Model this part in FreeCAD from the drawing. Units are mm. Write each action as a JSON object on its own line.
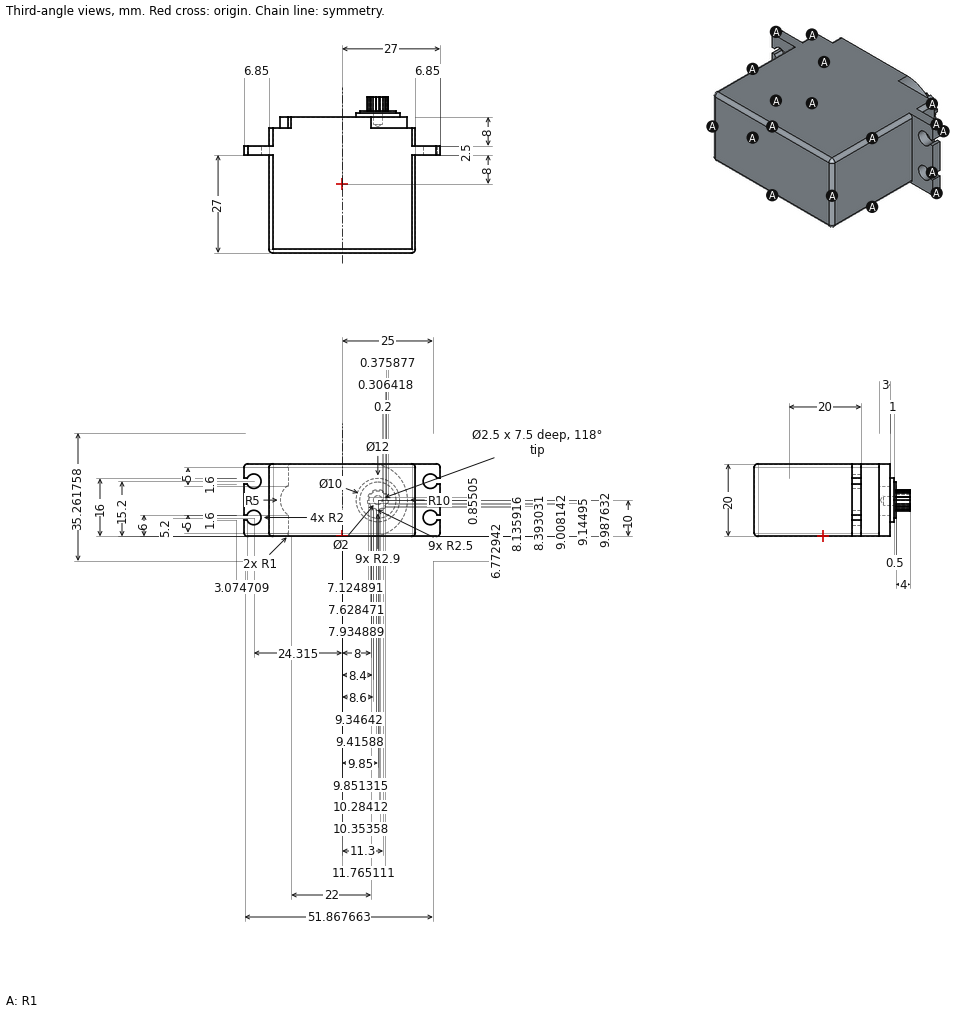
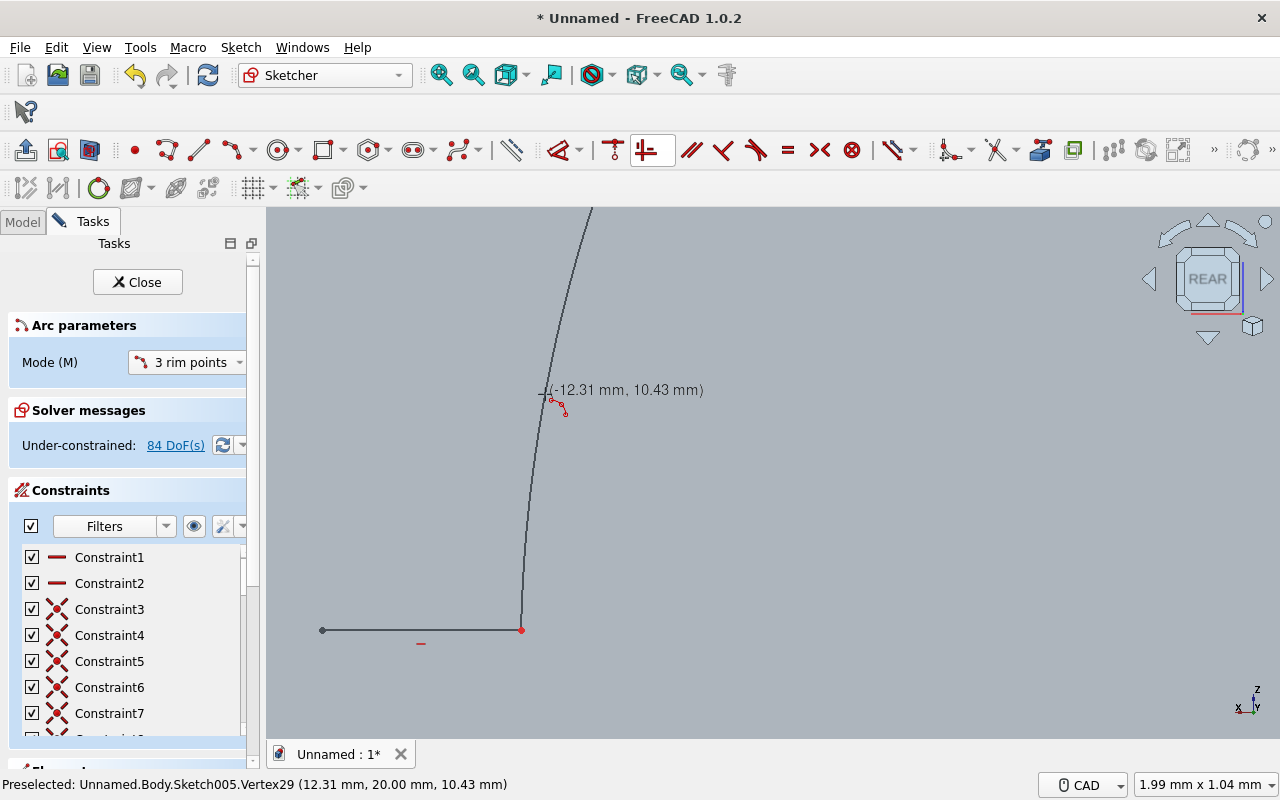
{"action": "scroll", "coordinate": [554, 370], "scroll_direction": "down", "scroll_amount": 15}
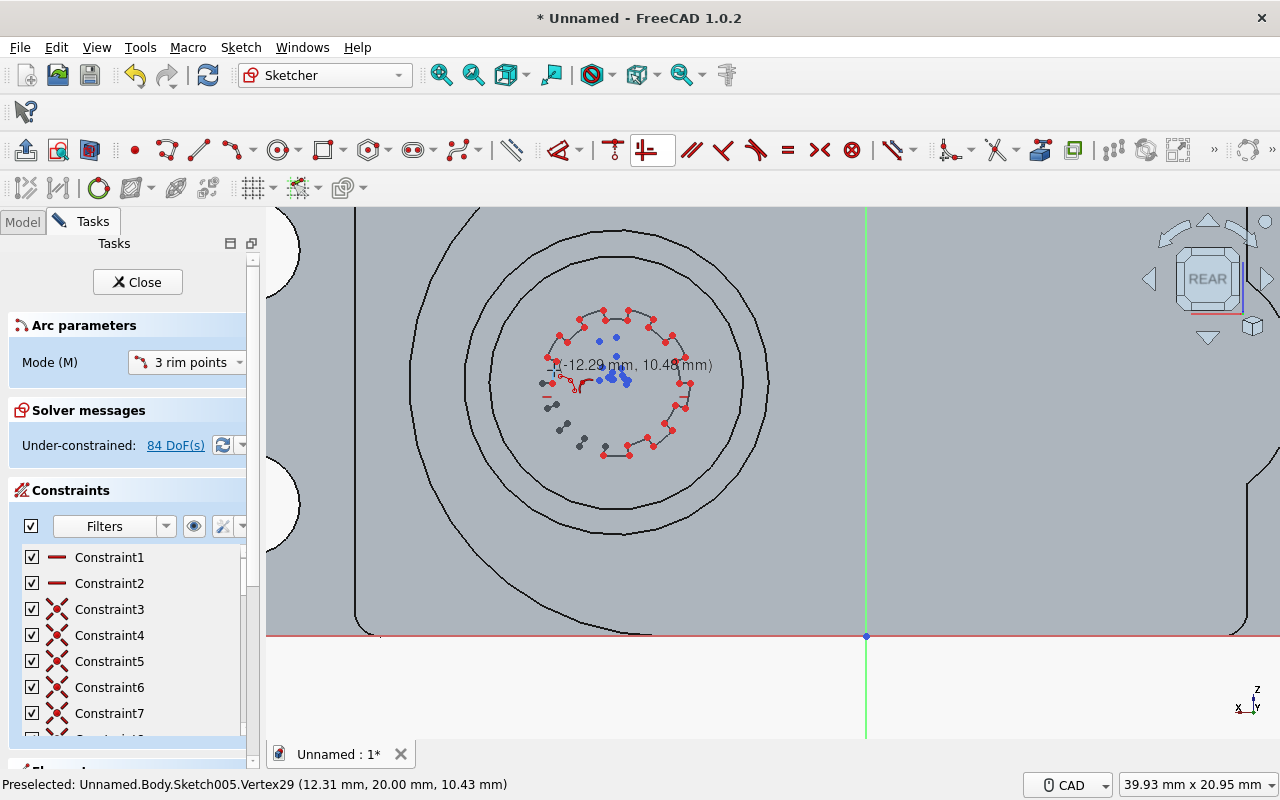
{"action": "scroll", "coordinate": [543, 383], "scroll_direction": "up", "scroll_amount": 6}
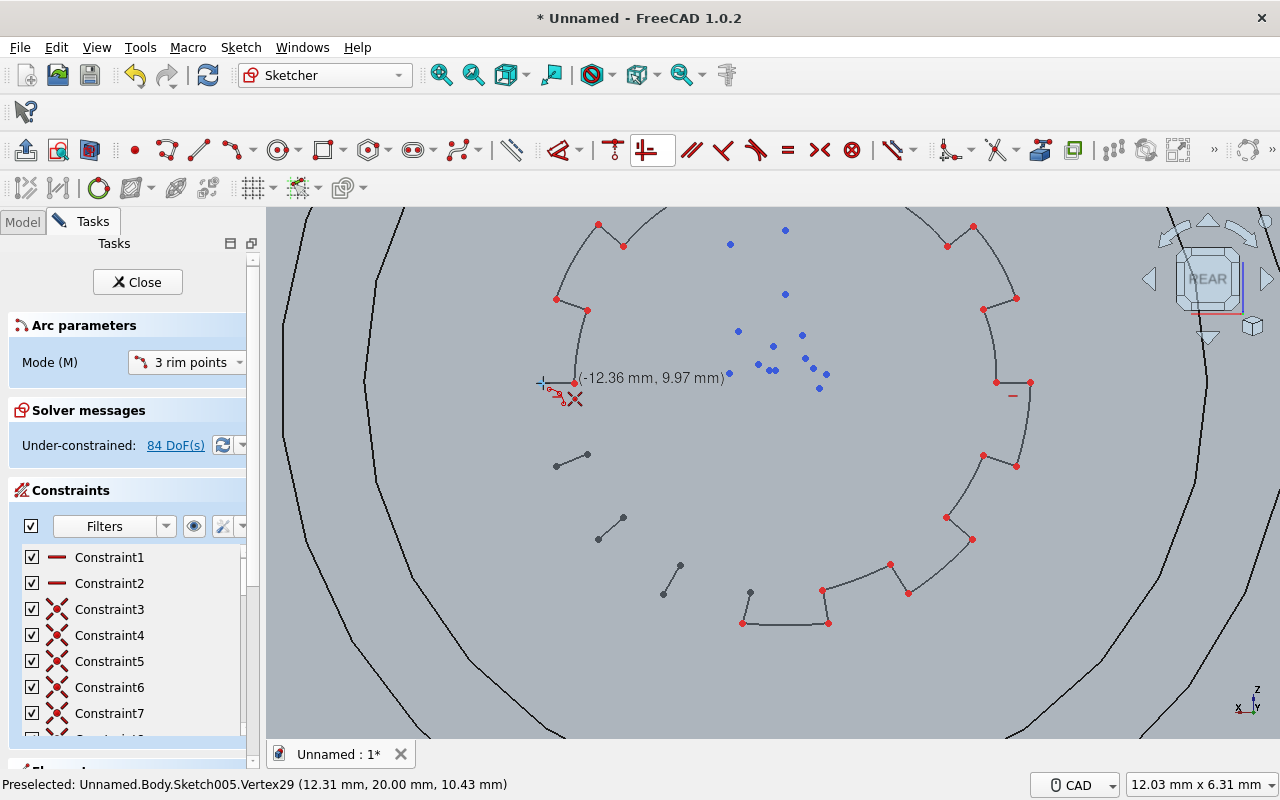
{"action": "left_click", "coordinate": [542, 383]}
{"action": "left_click", "coordinate": [556, 467]}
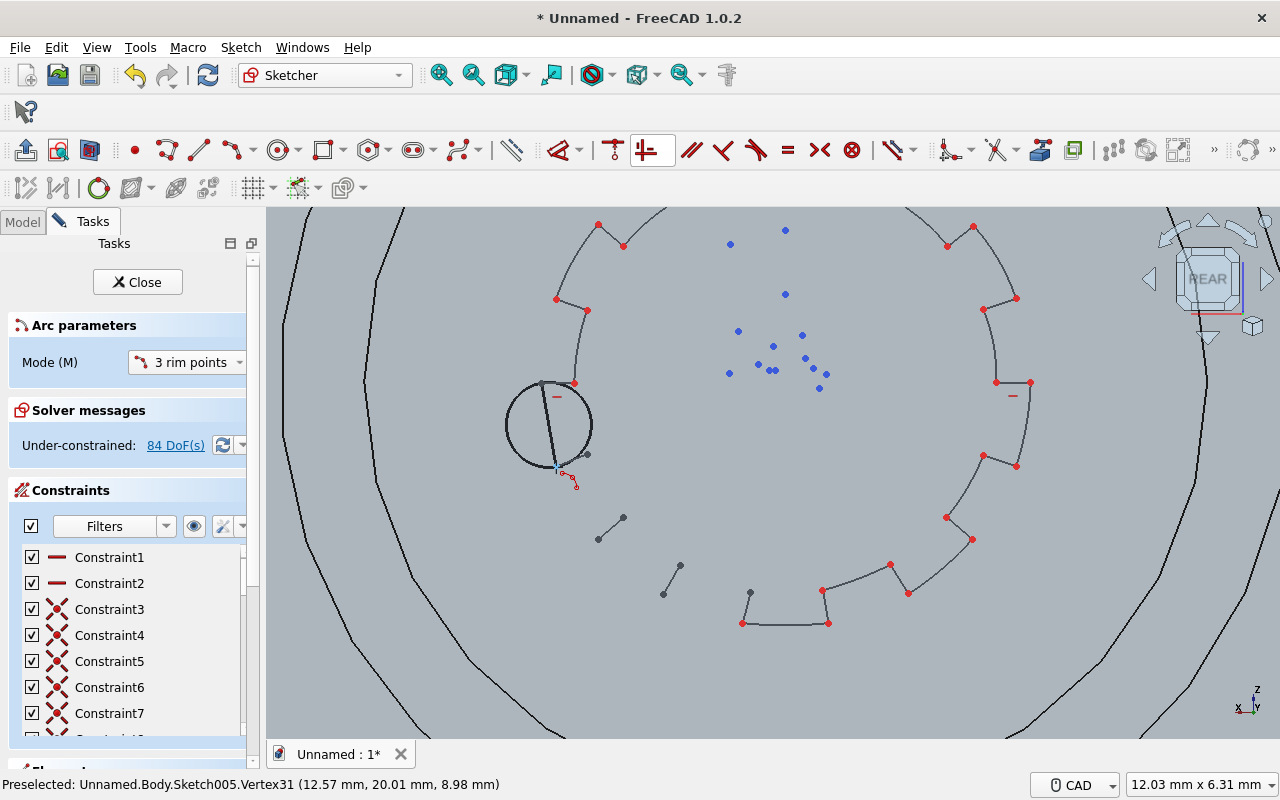
{"action": "scroll", "coordinate": [545, 423], "scroll_direction": "up", "scroll_amount": 8}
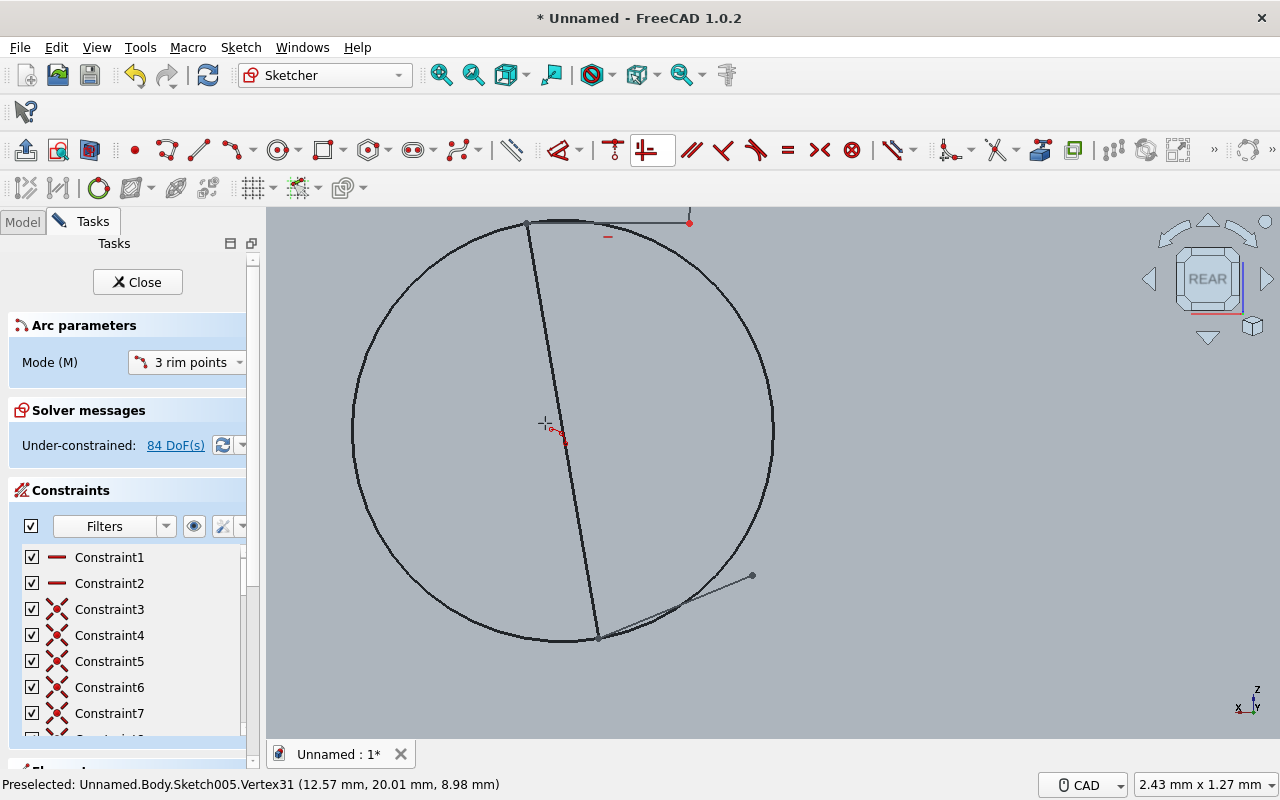
{"action": "left_click", "coordinate": [544, 422]}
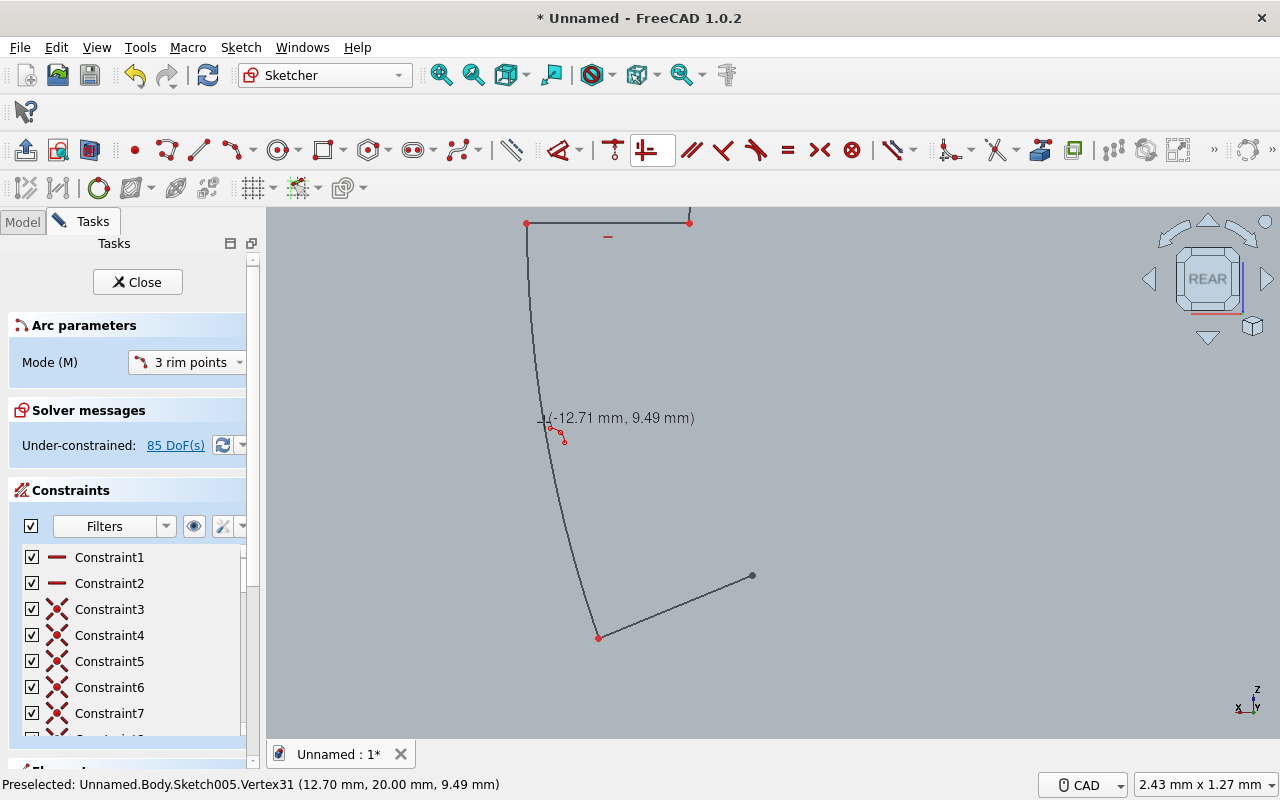
{"action": "scroll", "coordinate": [544, 393], "scroll_direction": "down", "scroll_amount": 14}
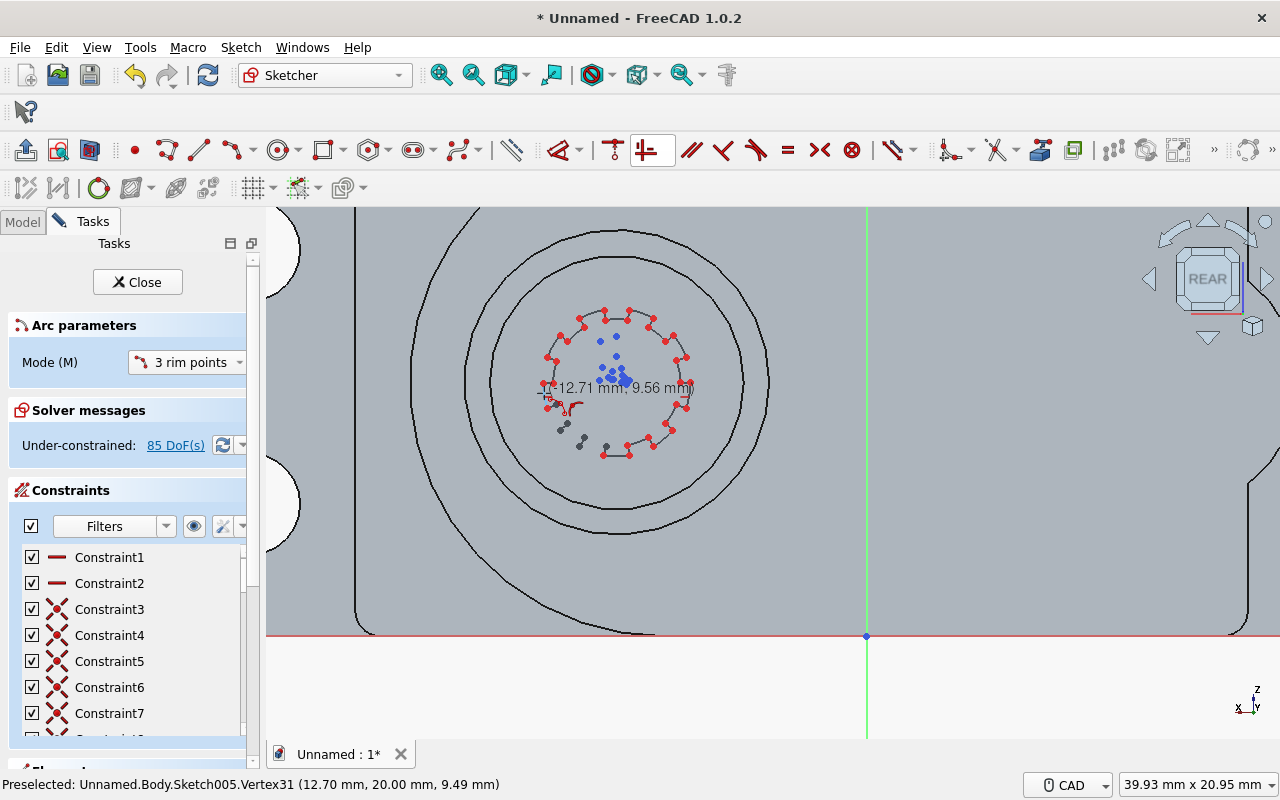
{"action": "scroll", "coordinate": [557, 404], "scroll_direction": "up", "scroll_amount": 6}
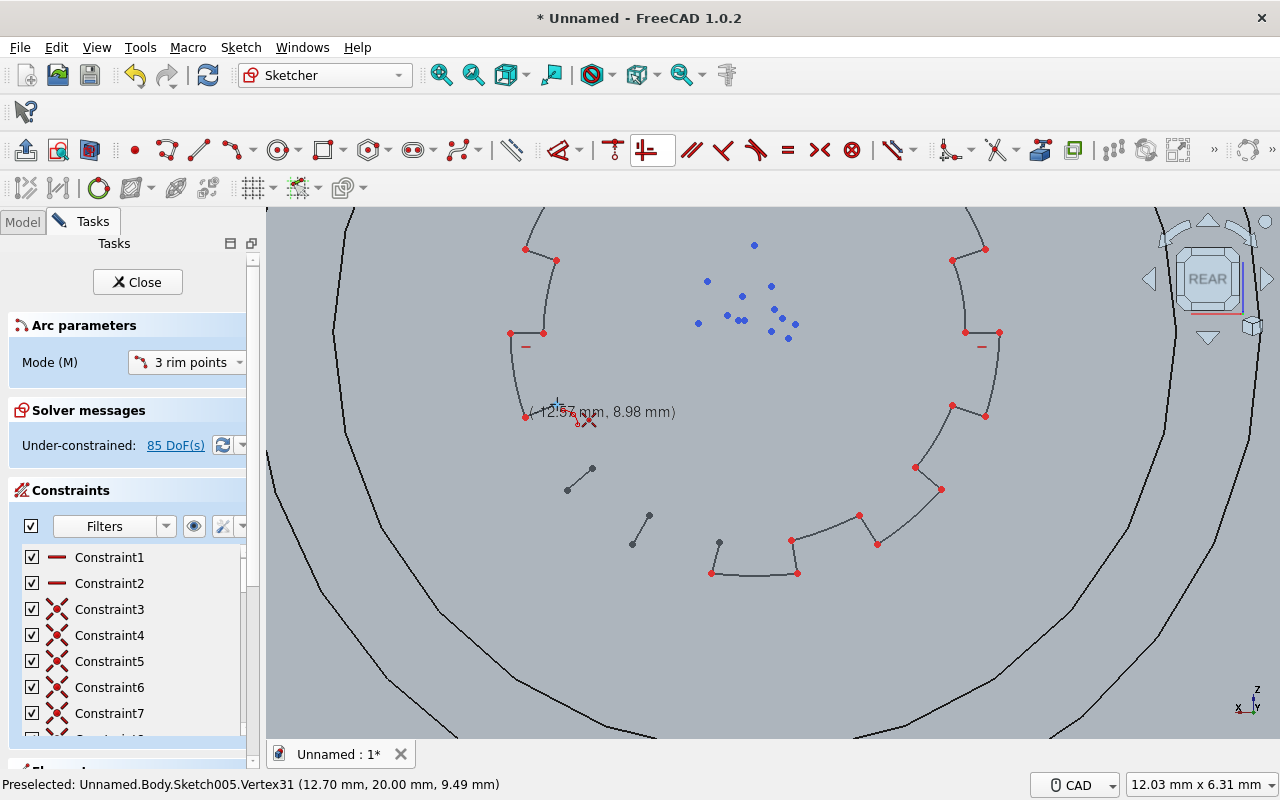
{"action": "left_click", "coordinate": [556, 405]}
{"action": "left_click", "coordinate": [593, 468]}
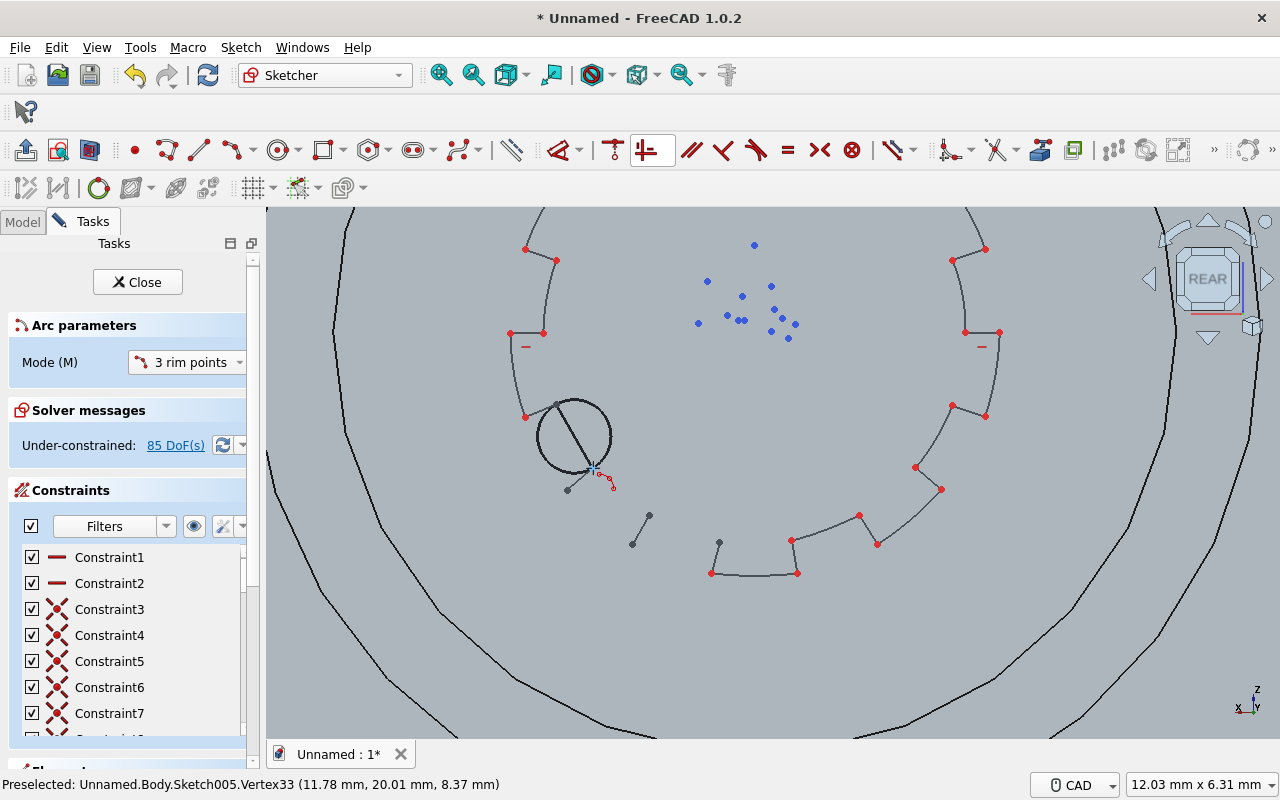
{"action": "scroll", "coordinate": [572, 436], "scroll_direction": "up", "scroll_amount": 9}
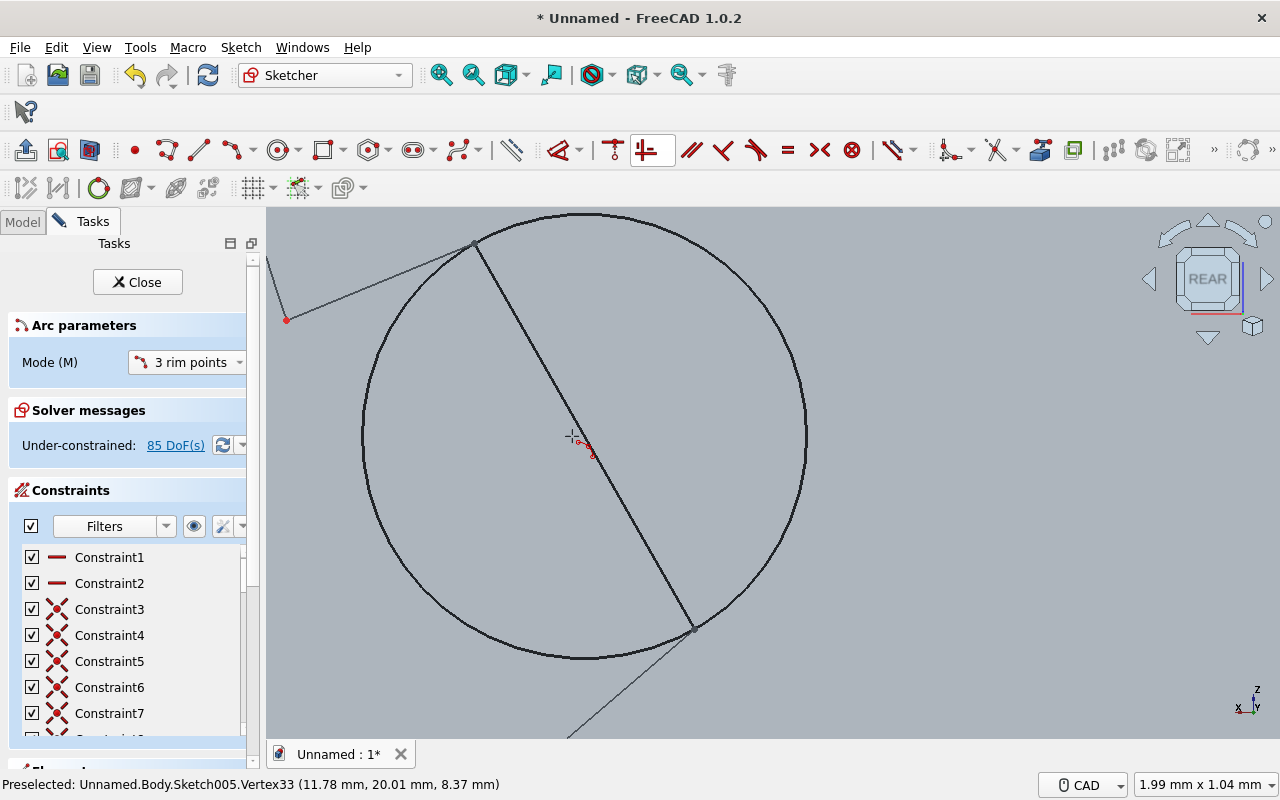
{"action": "left_click", "coordinate": [572, 436]}